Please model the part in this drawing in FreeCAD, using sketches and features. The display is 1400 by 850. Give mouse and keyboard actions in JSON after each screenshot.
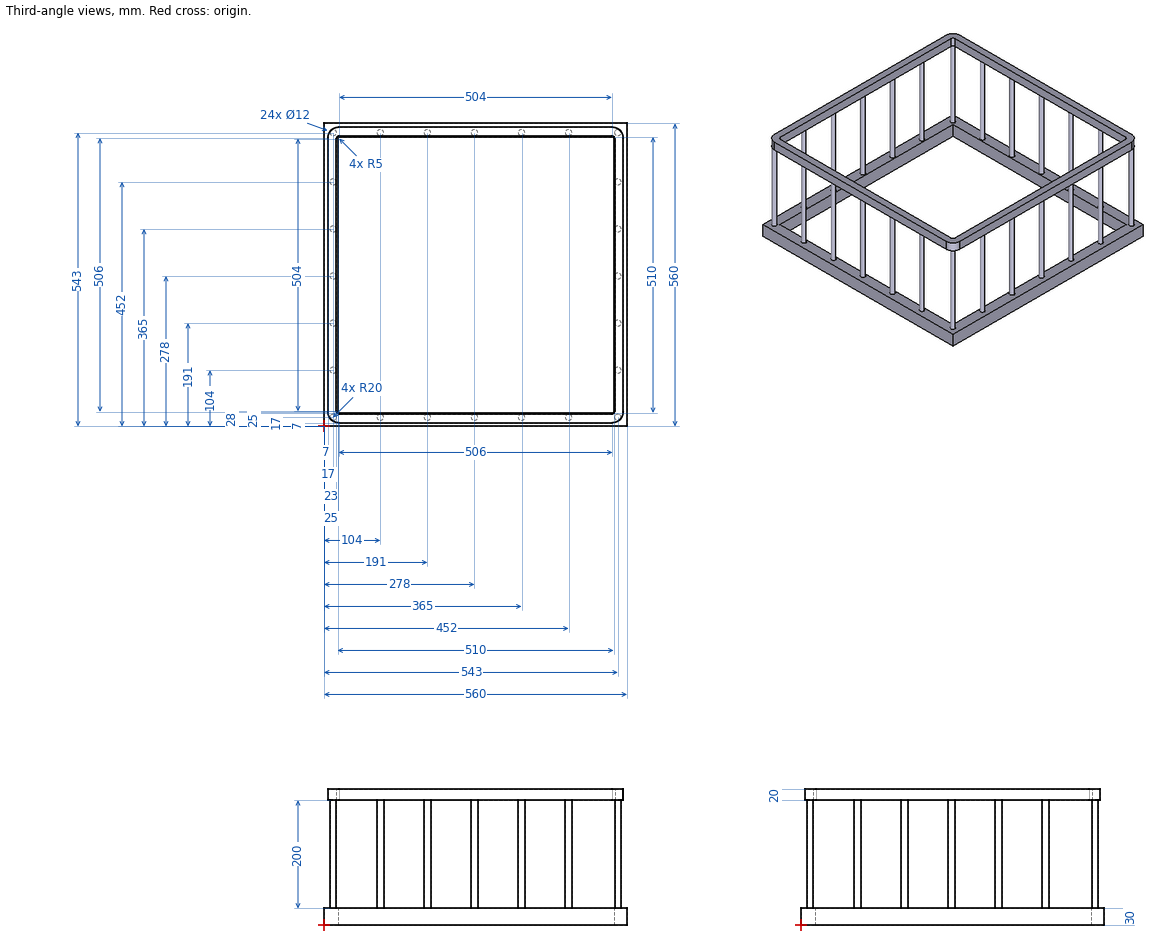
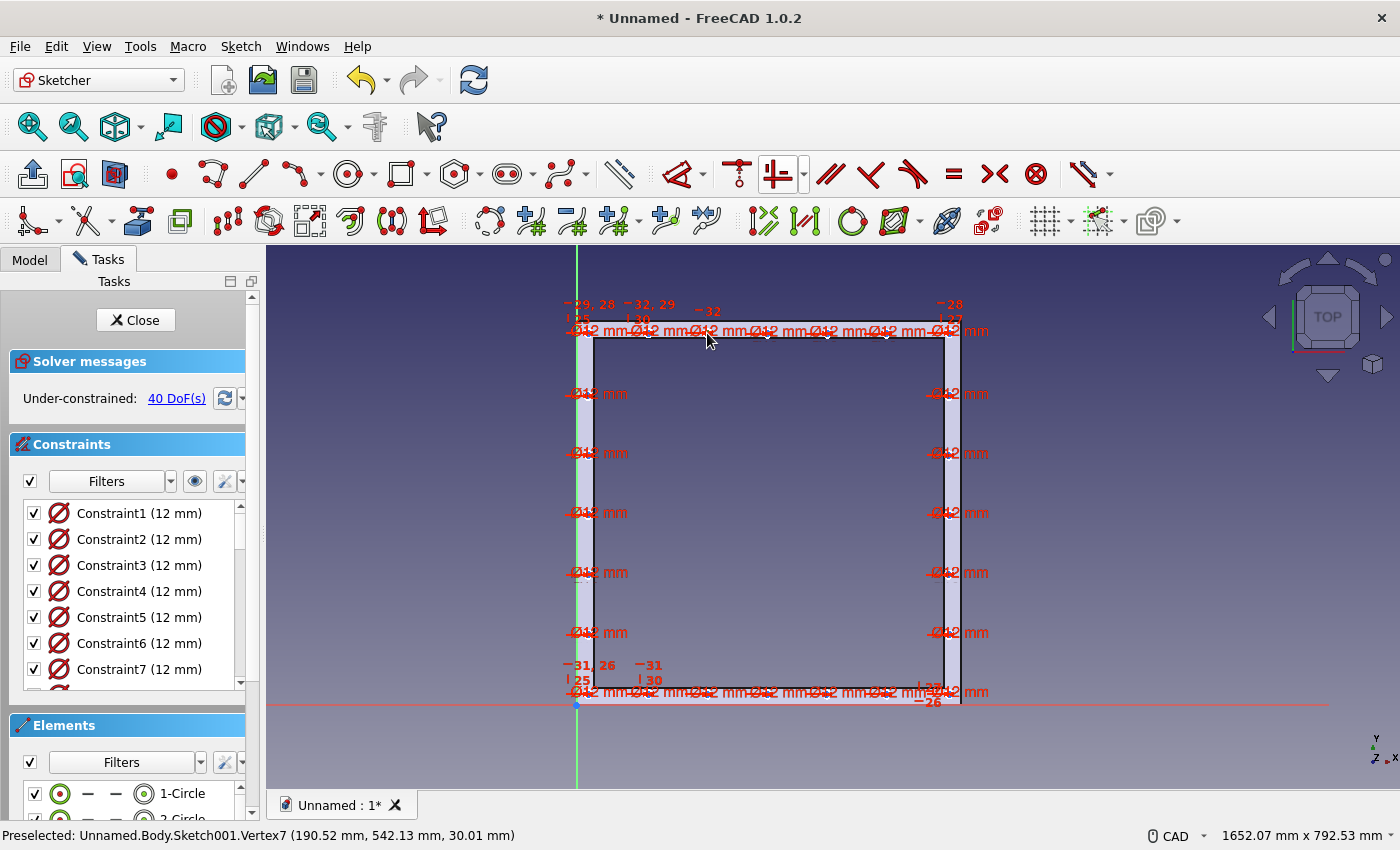
{"action": "left_click", "coordinate": [708, 694]}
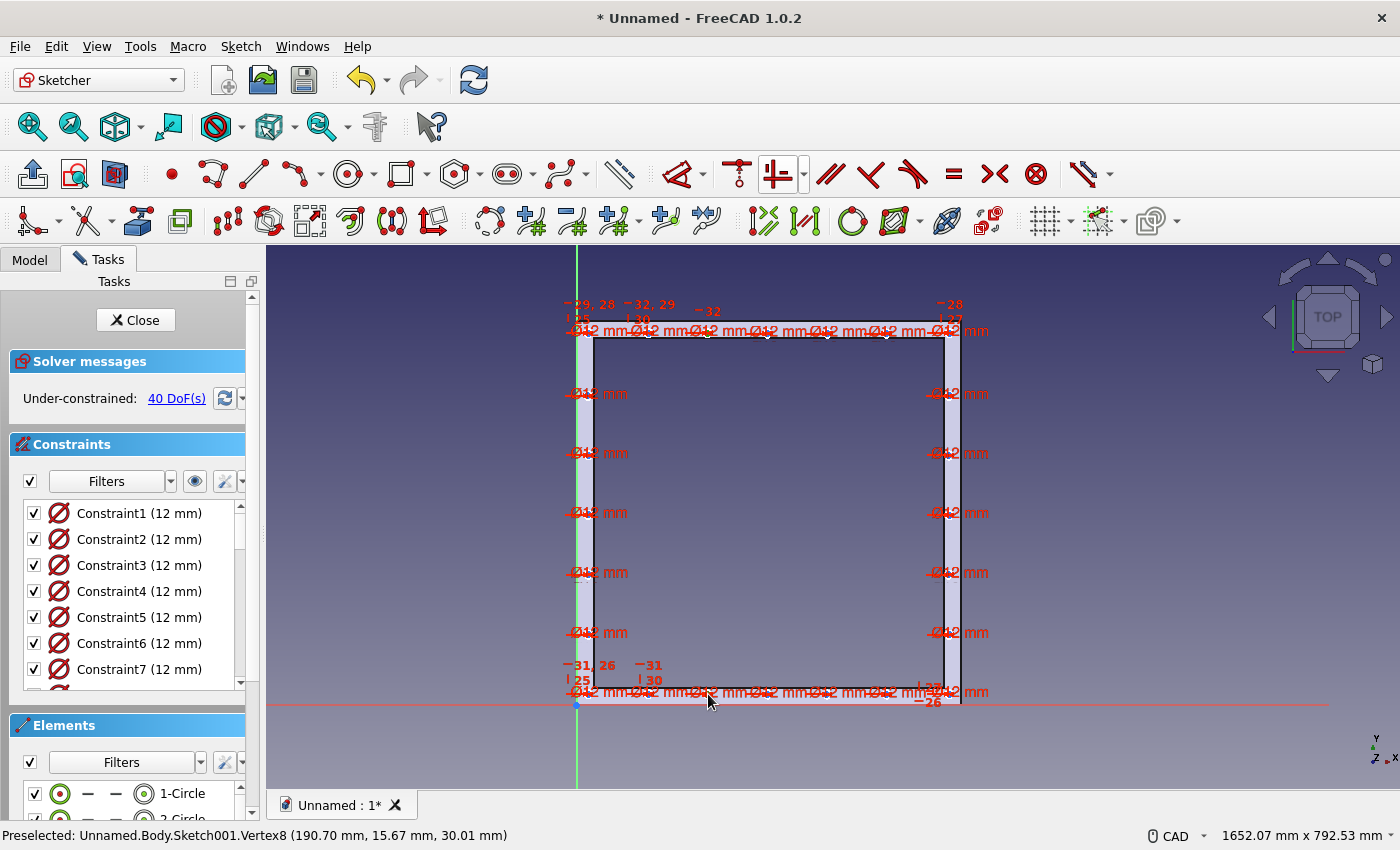
{"action": "key", "text": "v"}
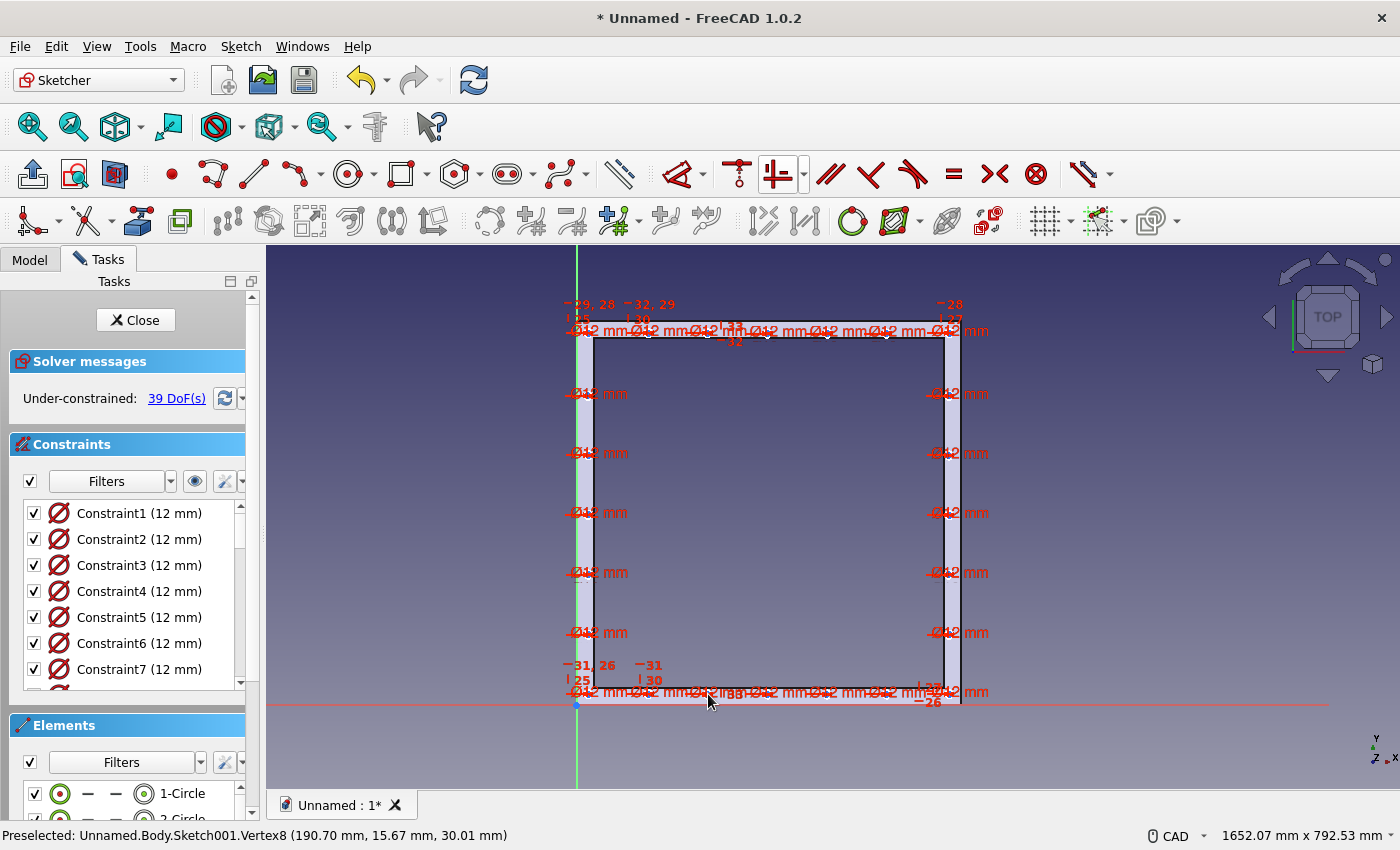
{"action": "left_click", "coordinate": [648, 694]}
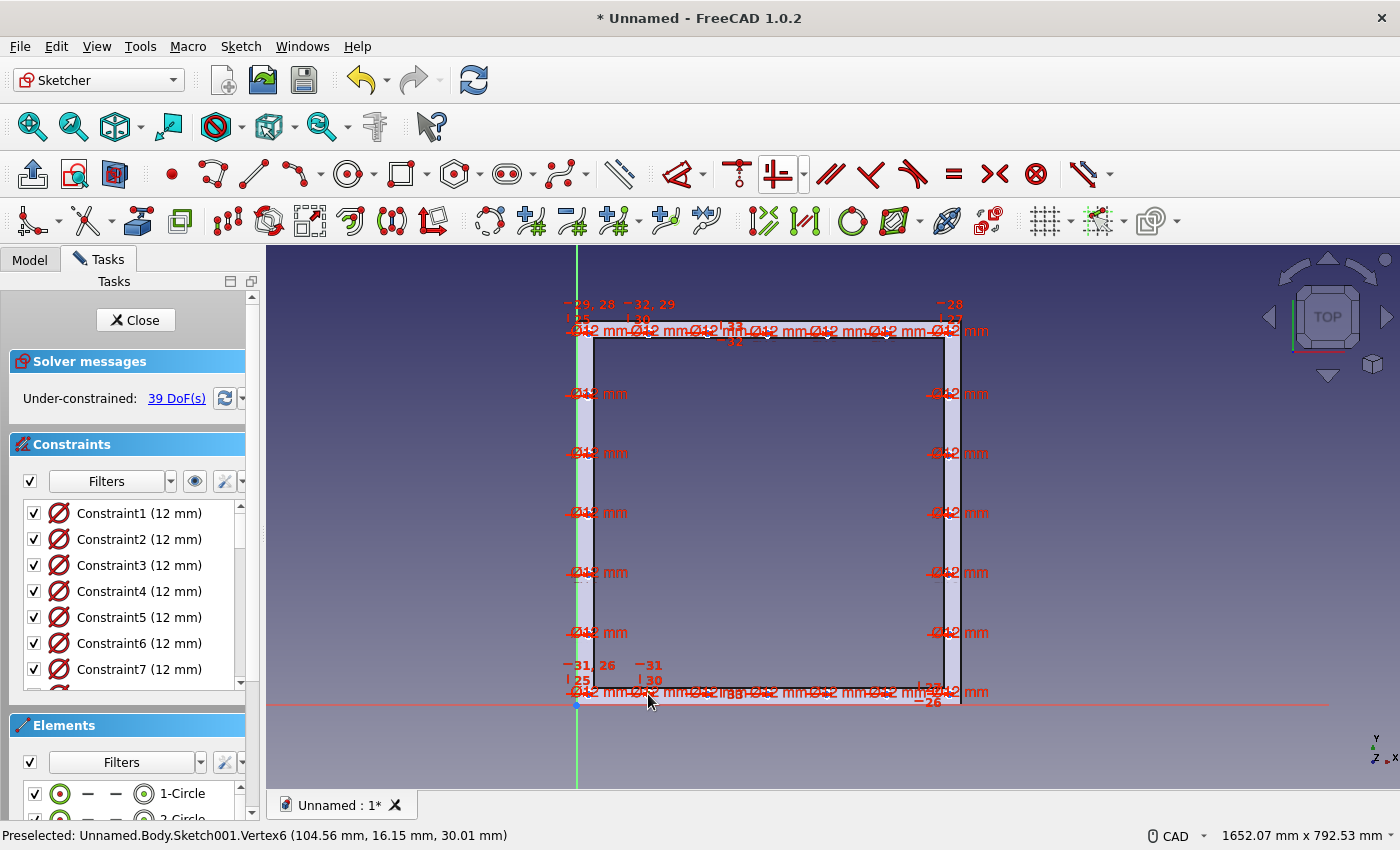
{"action": "left_click", "coordinate": [707, 694]}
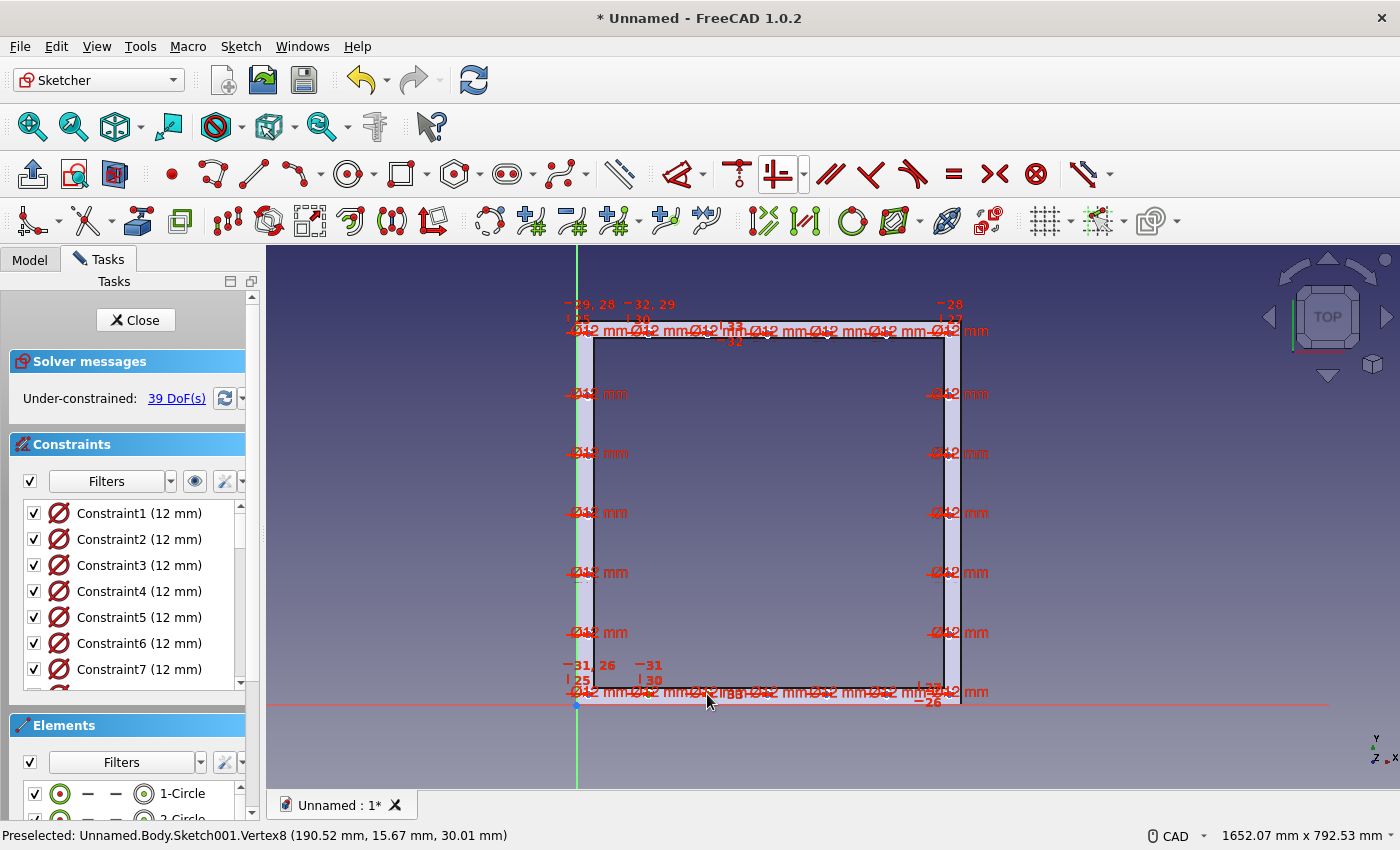
{"action": "left_click", "coordinate": [804, 174]}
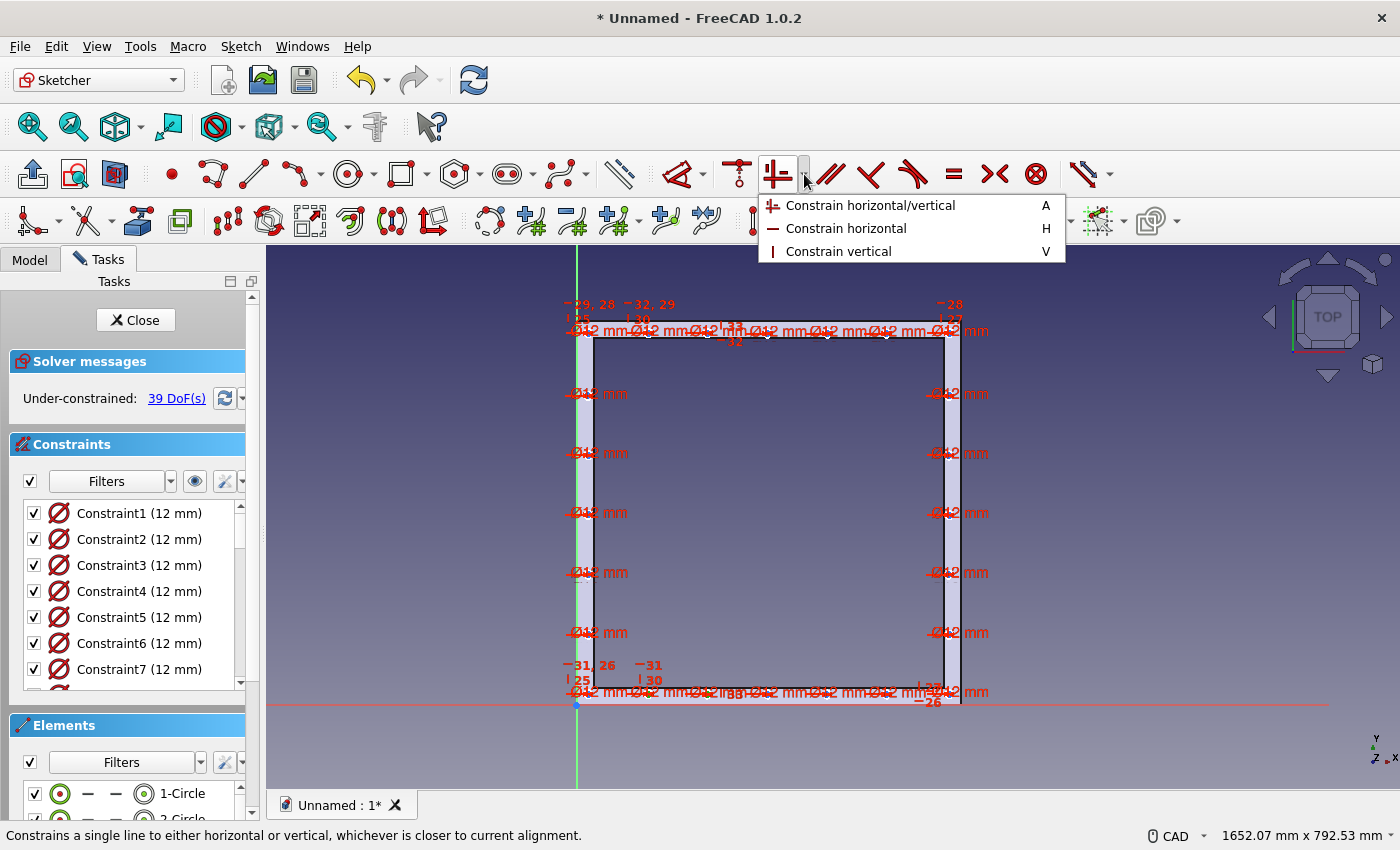
{"action": "left_click", "coordinate": [912, 228]}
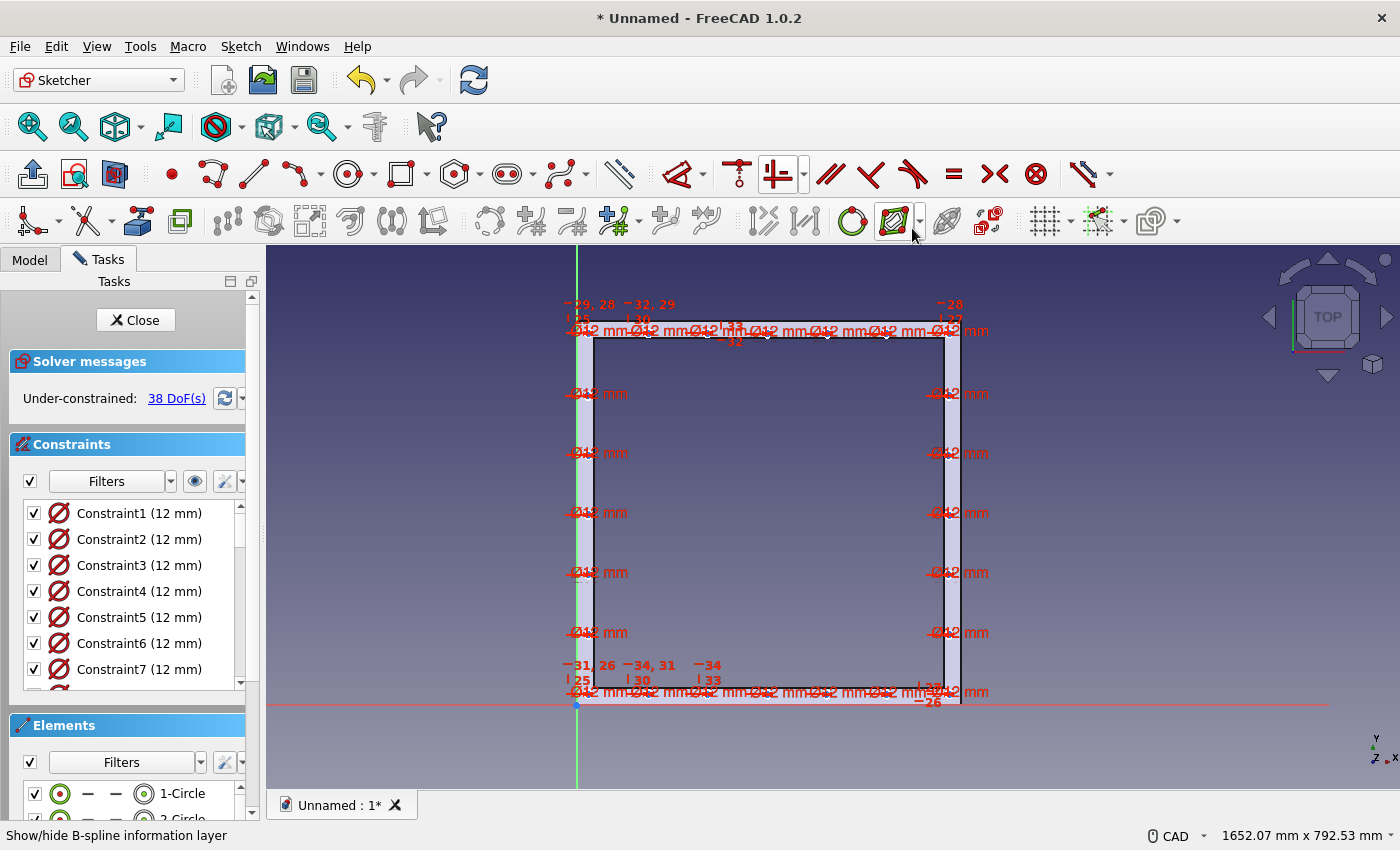
{"action": "left_click", "coordinate": [707, 333]}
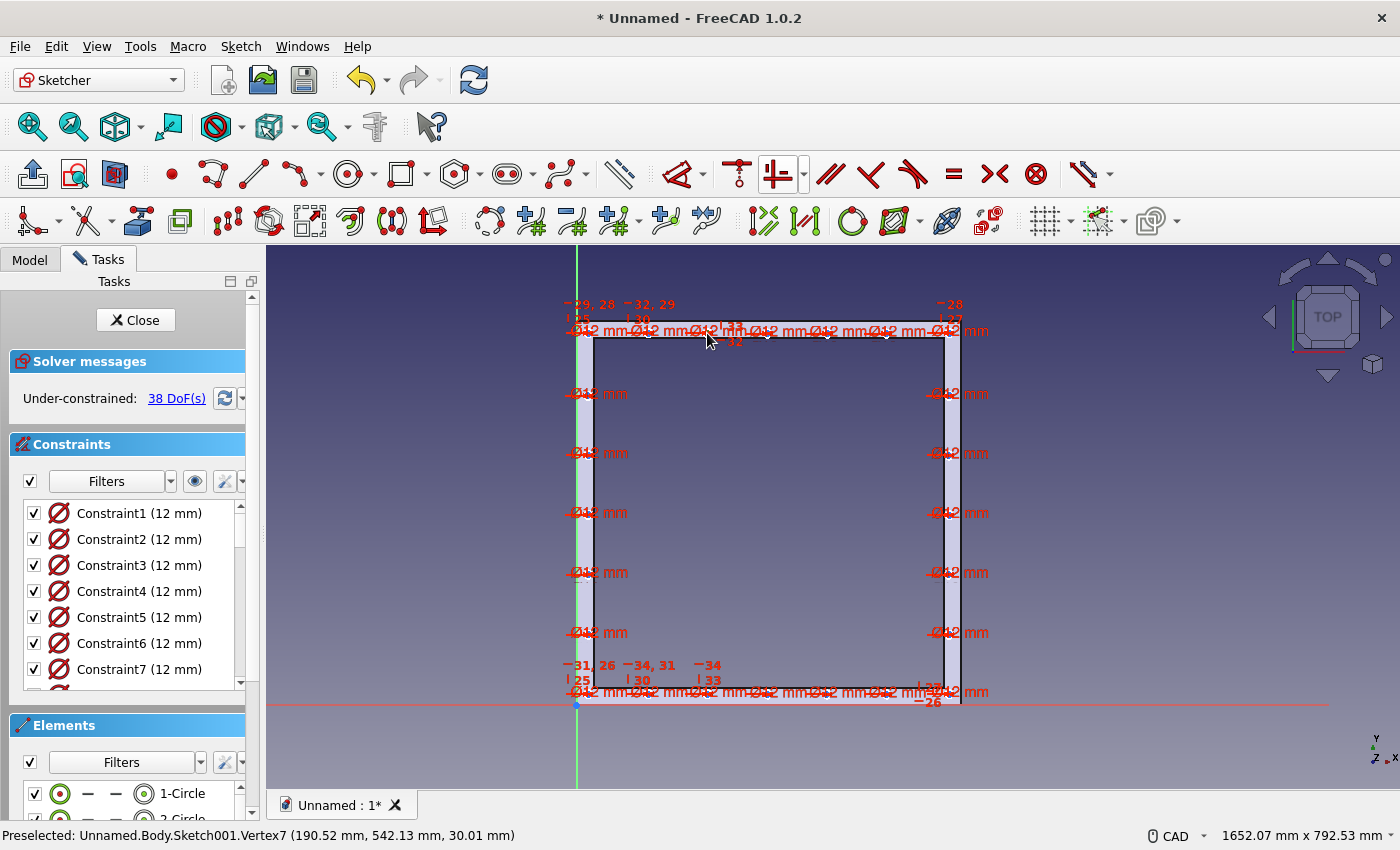
{"action": "left_click", "coordinate": [767, 334]}